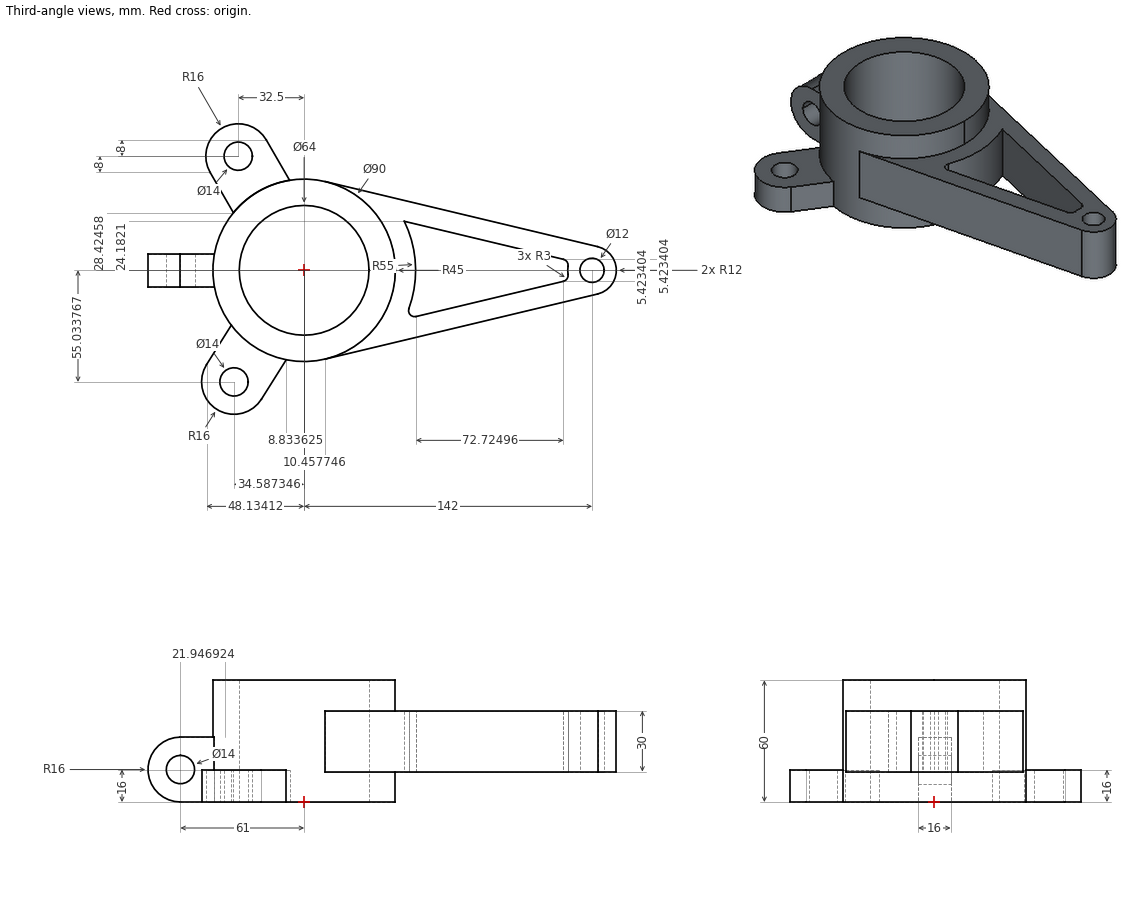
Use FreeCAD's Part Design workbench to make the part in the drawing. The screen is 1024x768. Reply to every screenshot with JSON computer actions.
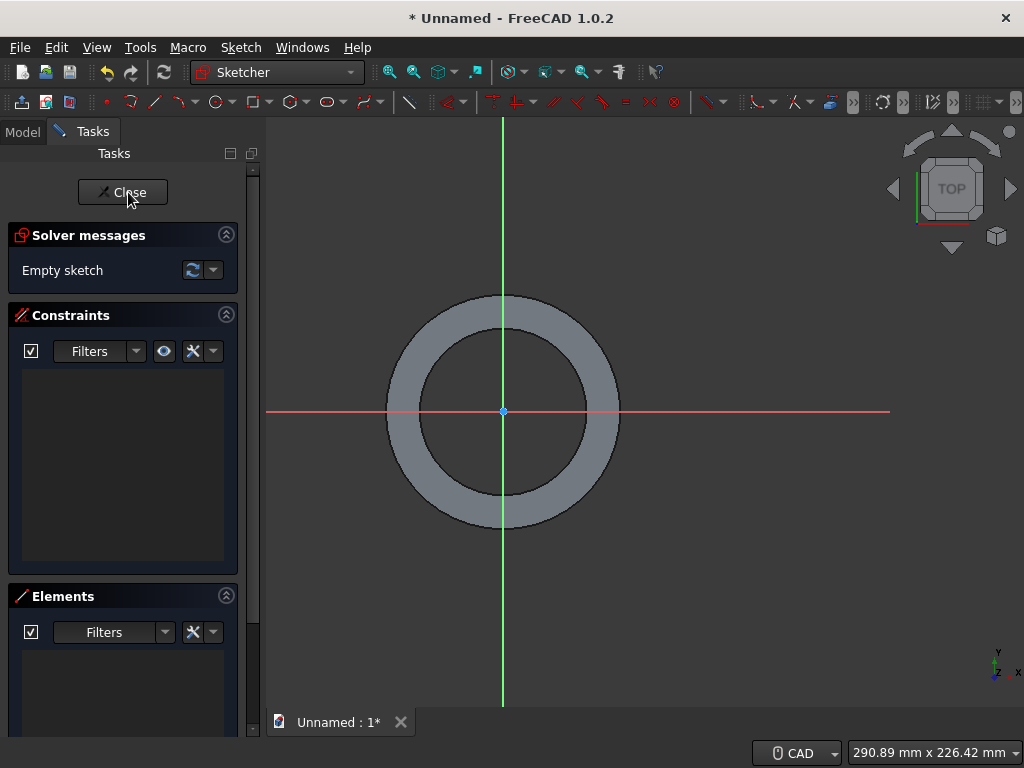
{"action": "scroll", "coordinate": [334, 246], "scroll_direction": "up", "scroll_amount": 4}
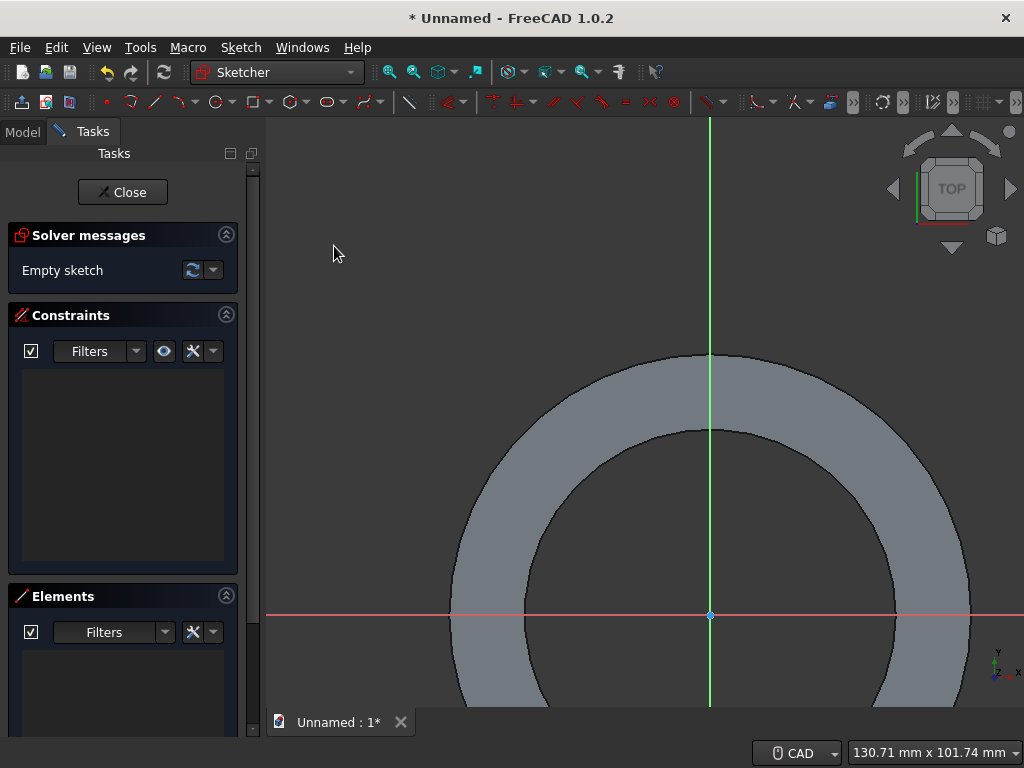
{"action": "key", "text": "g l"}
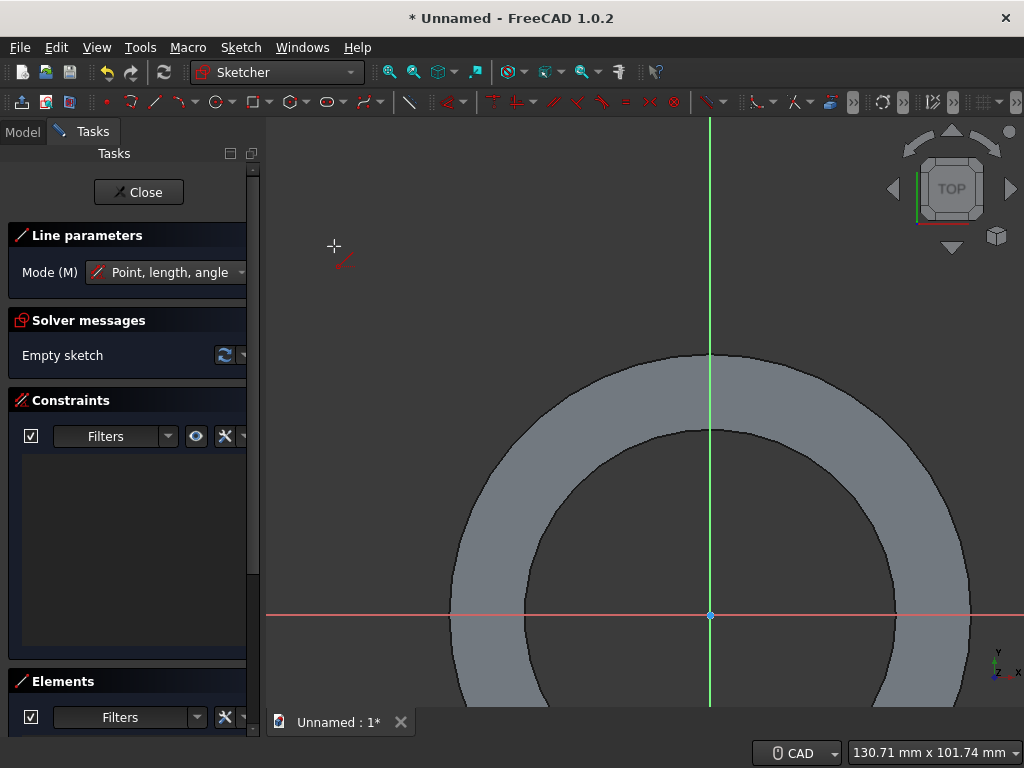
{"action": "left_click", "coordinate": [441, 335]}
{"action": "left_click", "coordinate": [508, 450]}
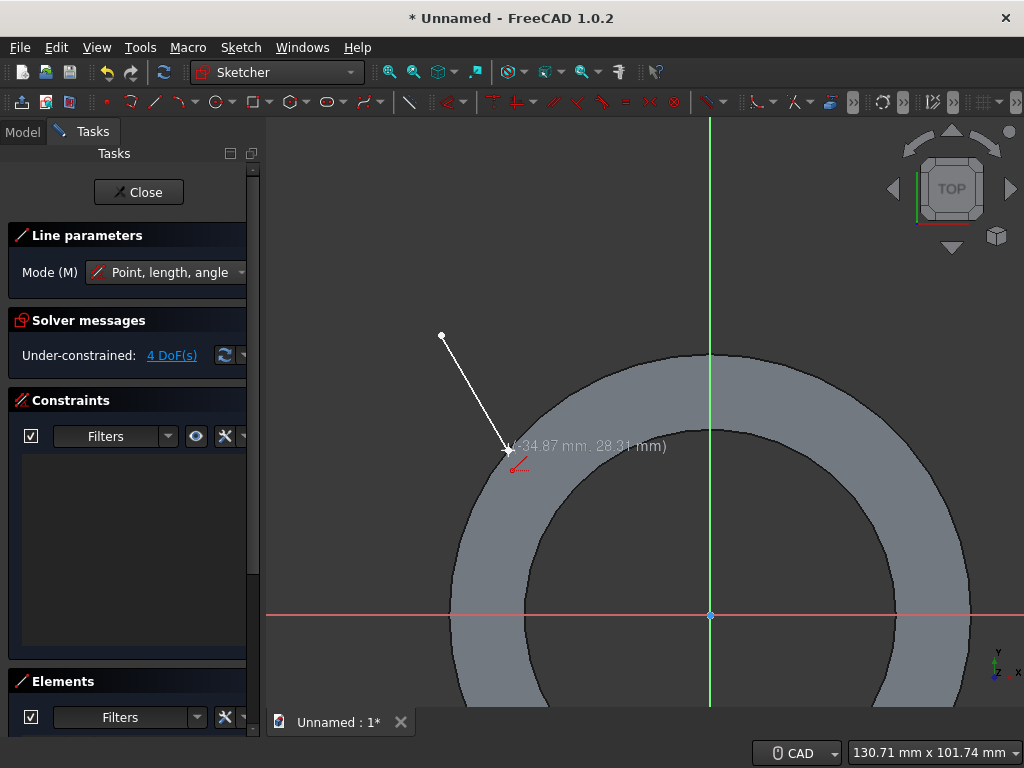
{"action": "left_click", "coordinate": [669, 358]}
{"action": "left_click", "coordinate": [602, 242]}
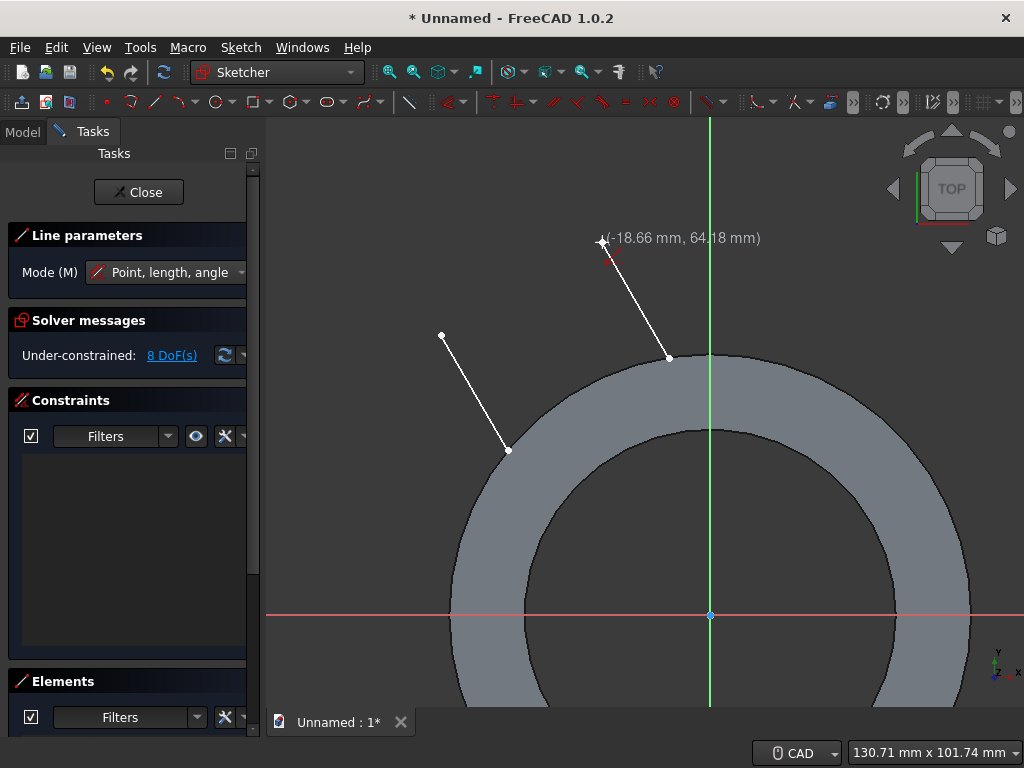
{"action": "key", "text": "g 3 a"}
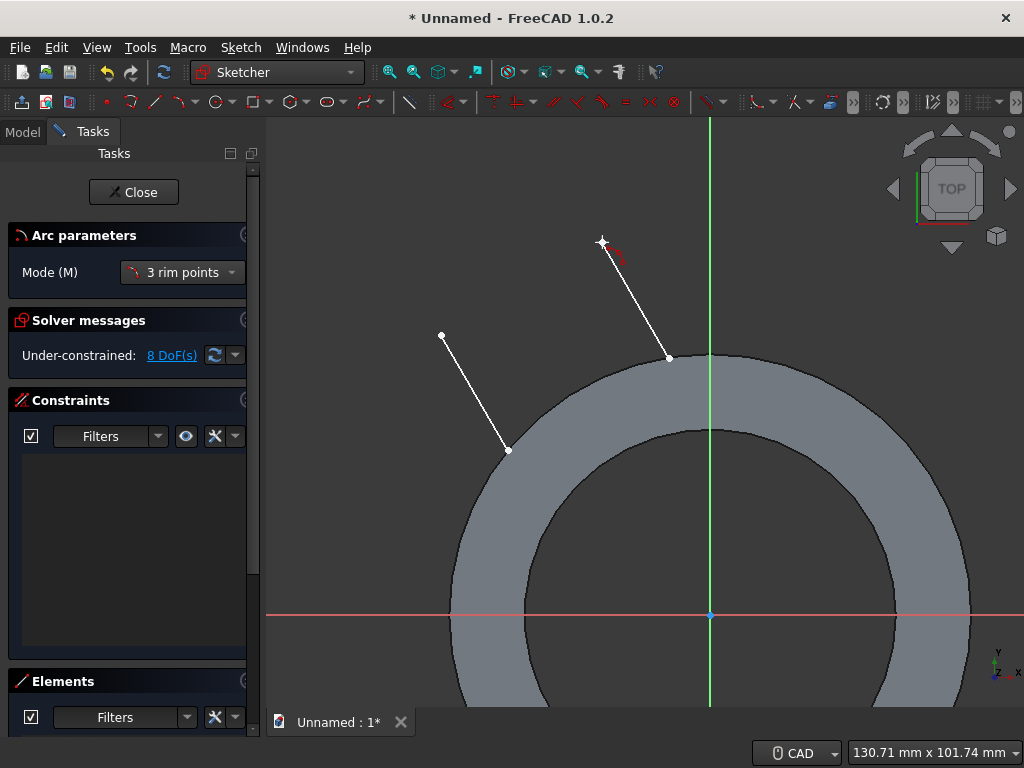
{"action": "left_click", "coordinate": [508, 451]}
{"action": "left_click", "coordinate": [669, 359]}
{"action": "left_click", "coordinate": [580, 389]}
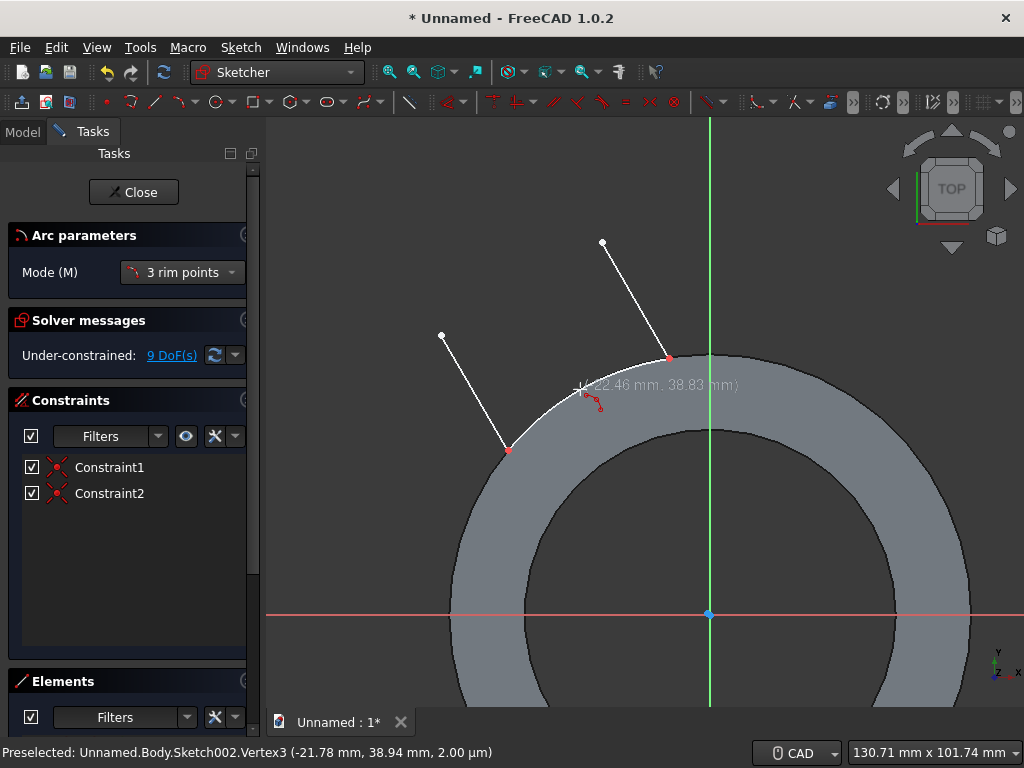
{"action": "left_click", "coordinate": [602, 243]}
{"action": "left_click", "coordinate": [441, 336]}
{"action": "left_click", "coordinate": [475, 208]}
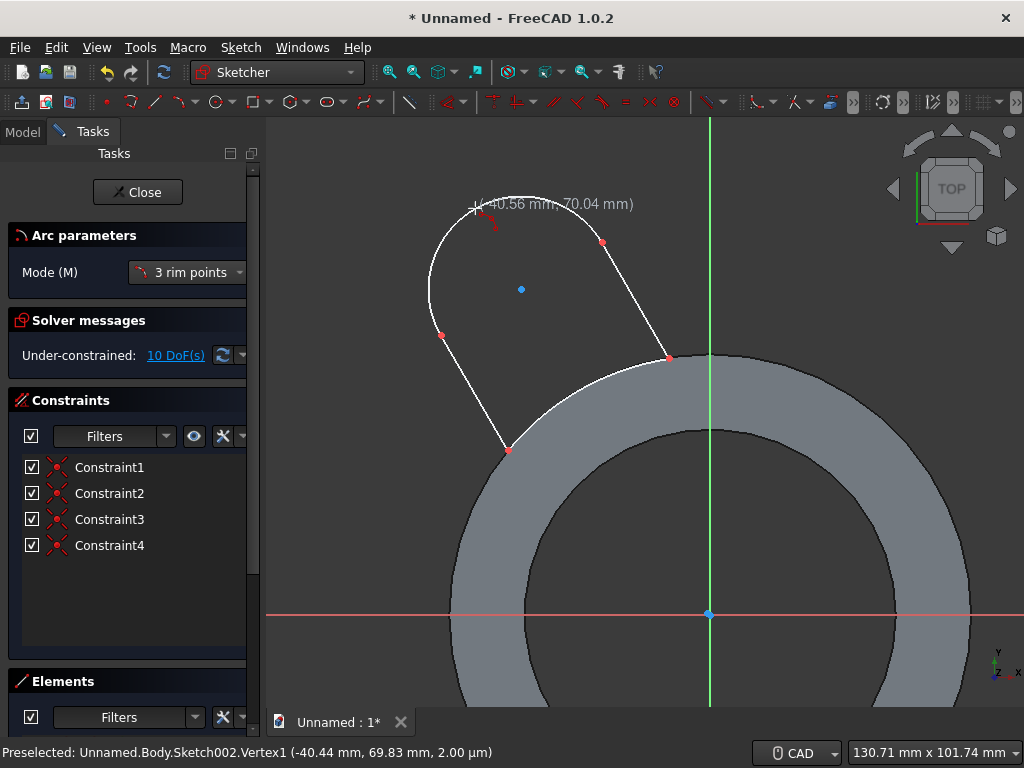
{"action": "left_click", "coordinate": [216, 102]}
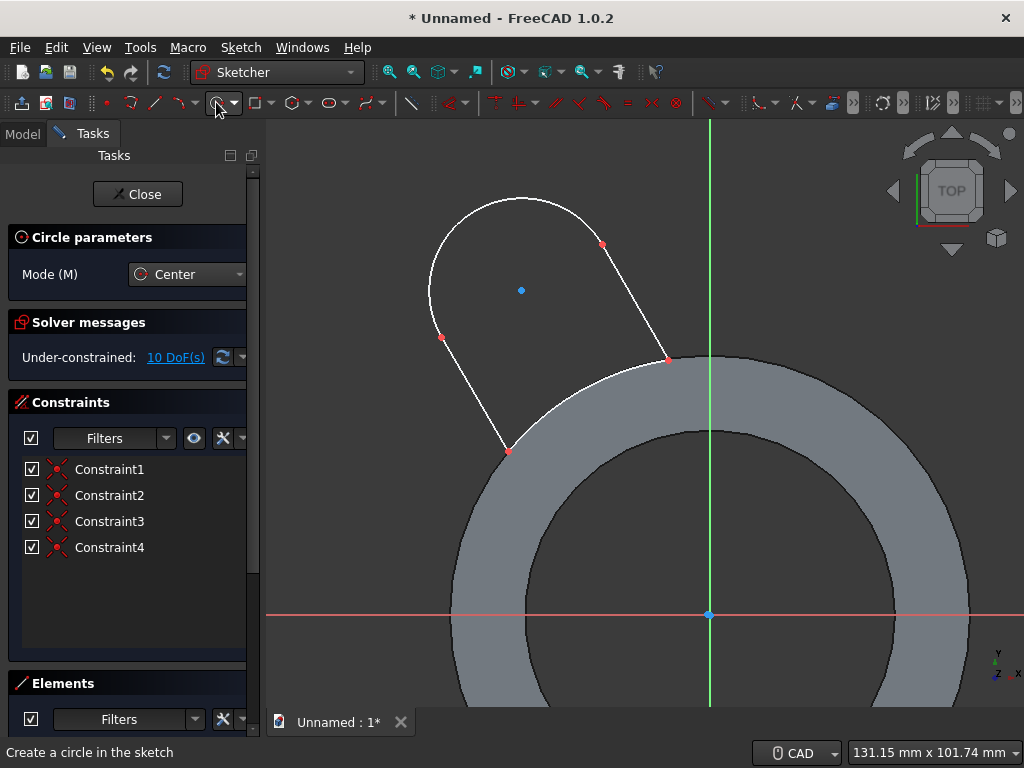
{"action": "left_click", "coordinate": [522, 290]}
{"action": "left_click", "coordinate": [551, 262]}
{"action": "key", "text": "Escape"}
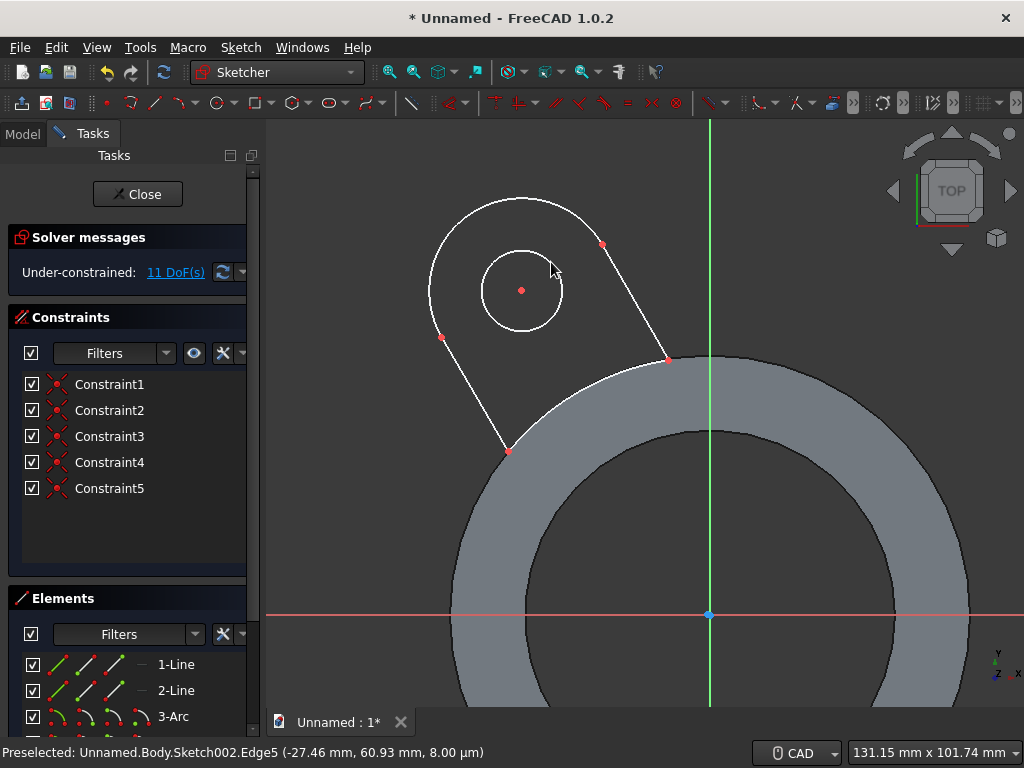
{"action": "left_click", "coordinate": [462, 372]}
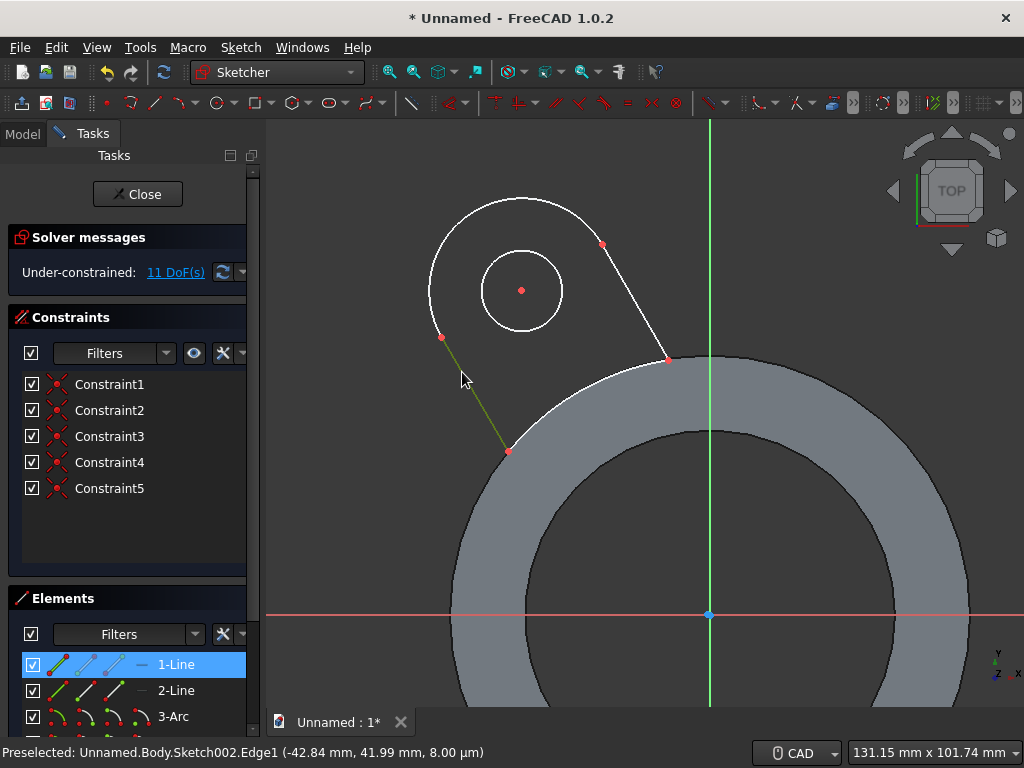
{"action": "left_click", "coordinate": [532, 199]}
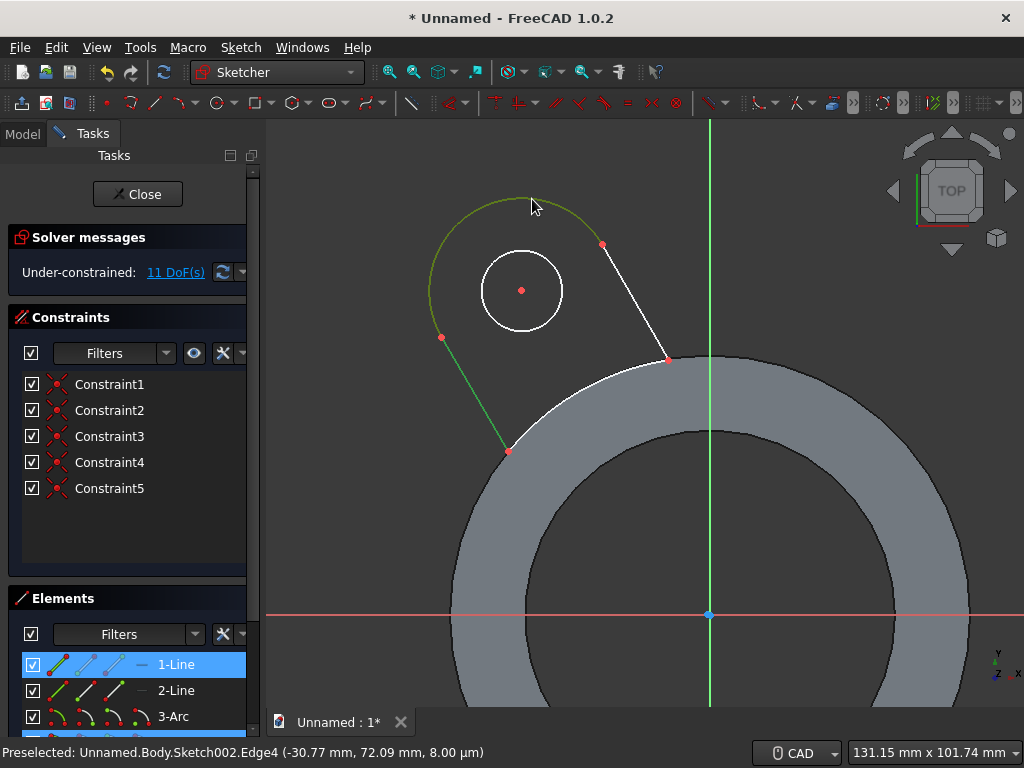
{"action": "left_click", "coordinate": [604, 104]}